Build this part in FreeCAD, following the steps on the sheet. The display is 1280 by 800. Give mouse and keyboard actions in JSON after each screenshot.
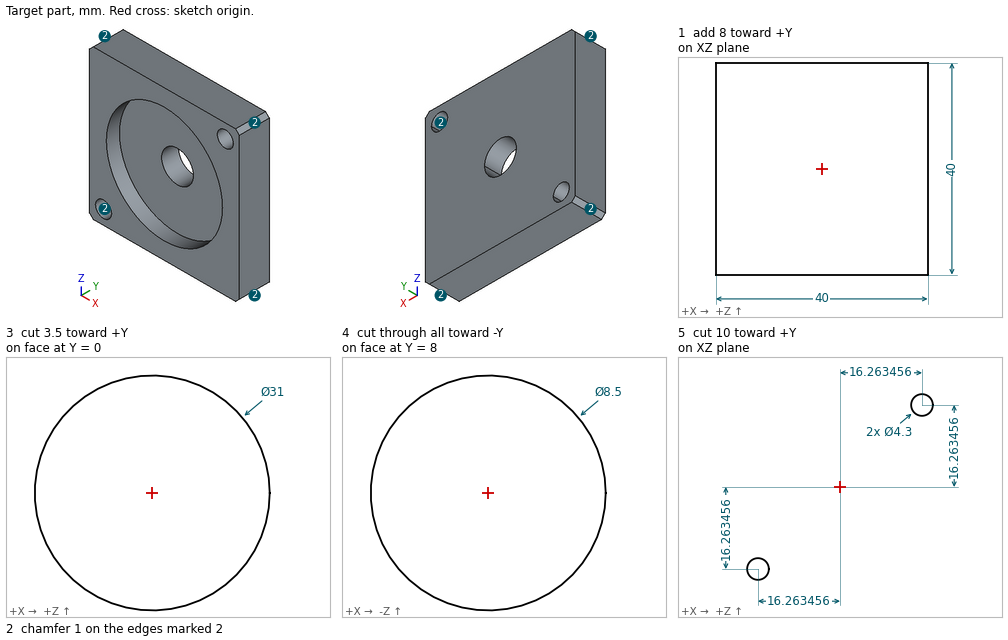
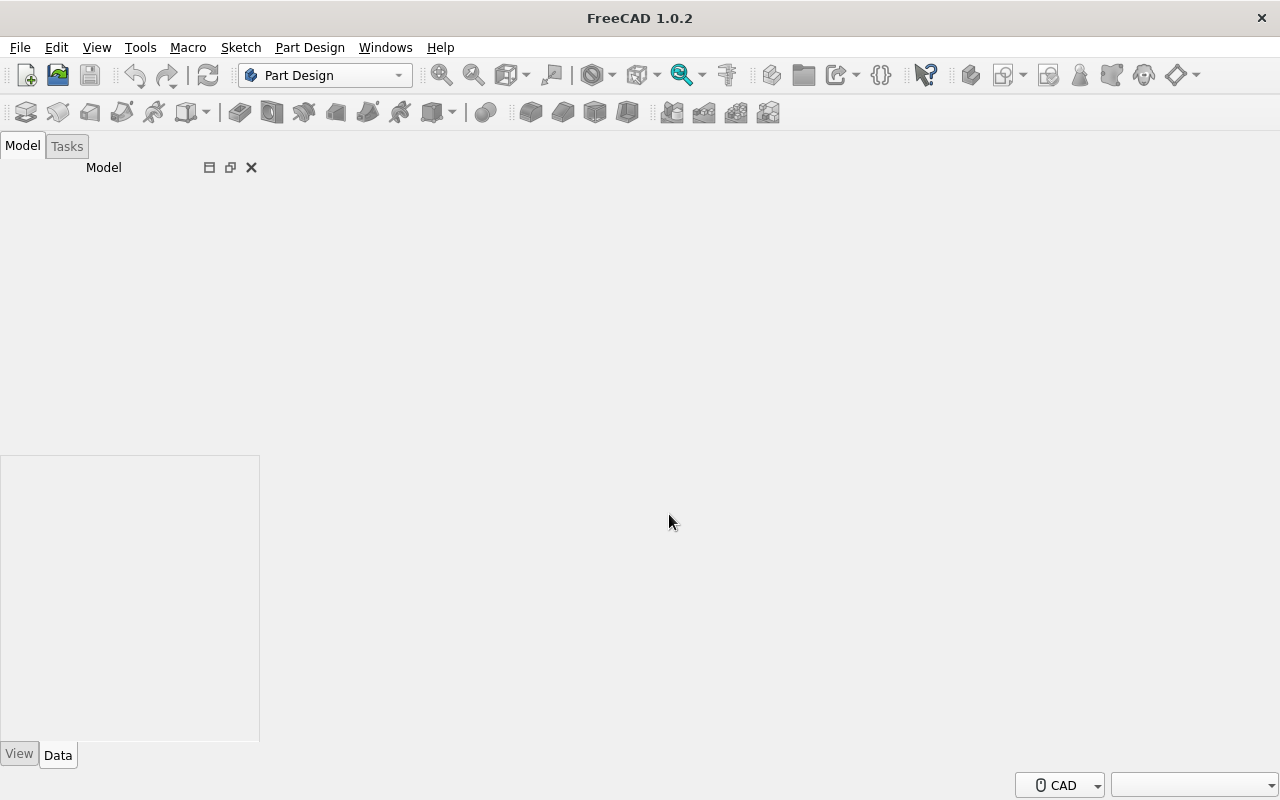
{"action": "left_click", "coordinate": [26, 76]}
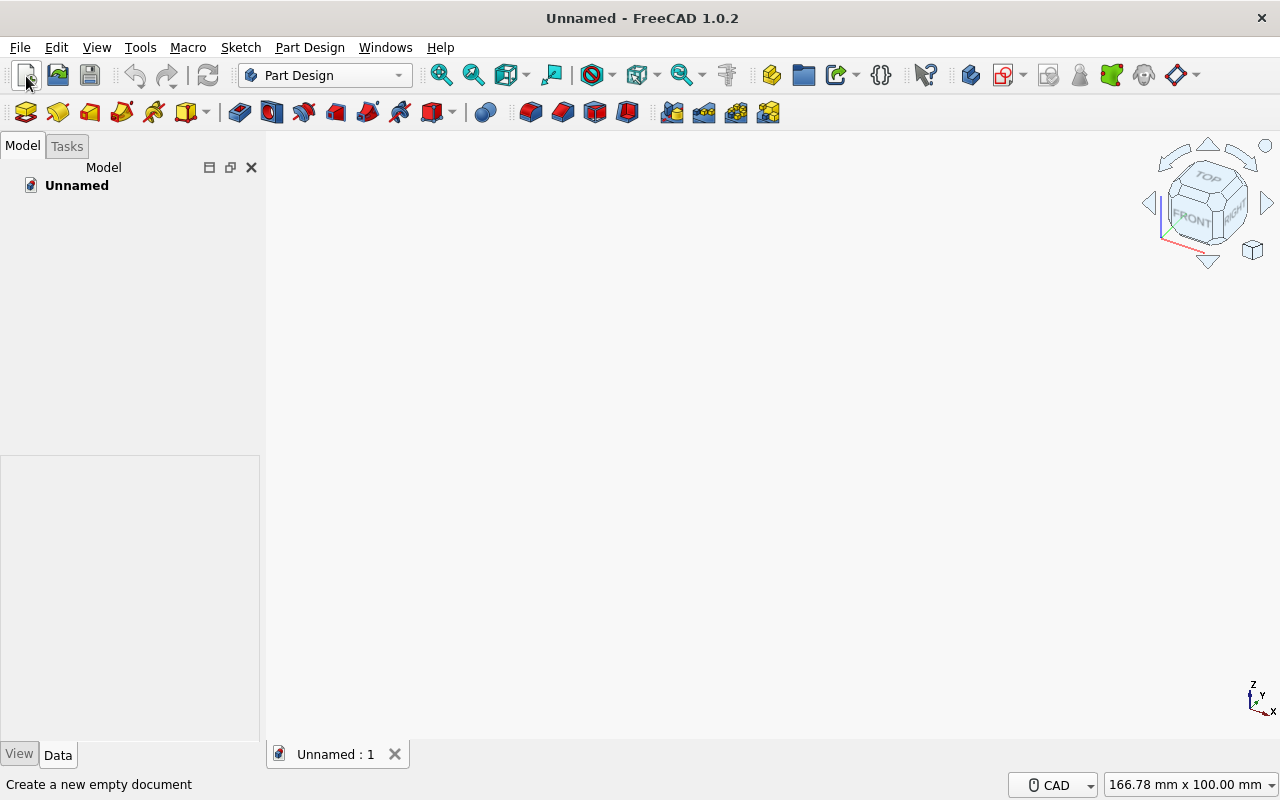
{"action": "left_click", "coordinate": [1004, 76]}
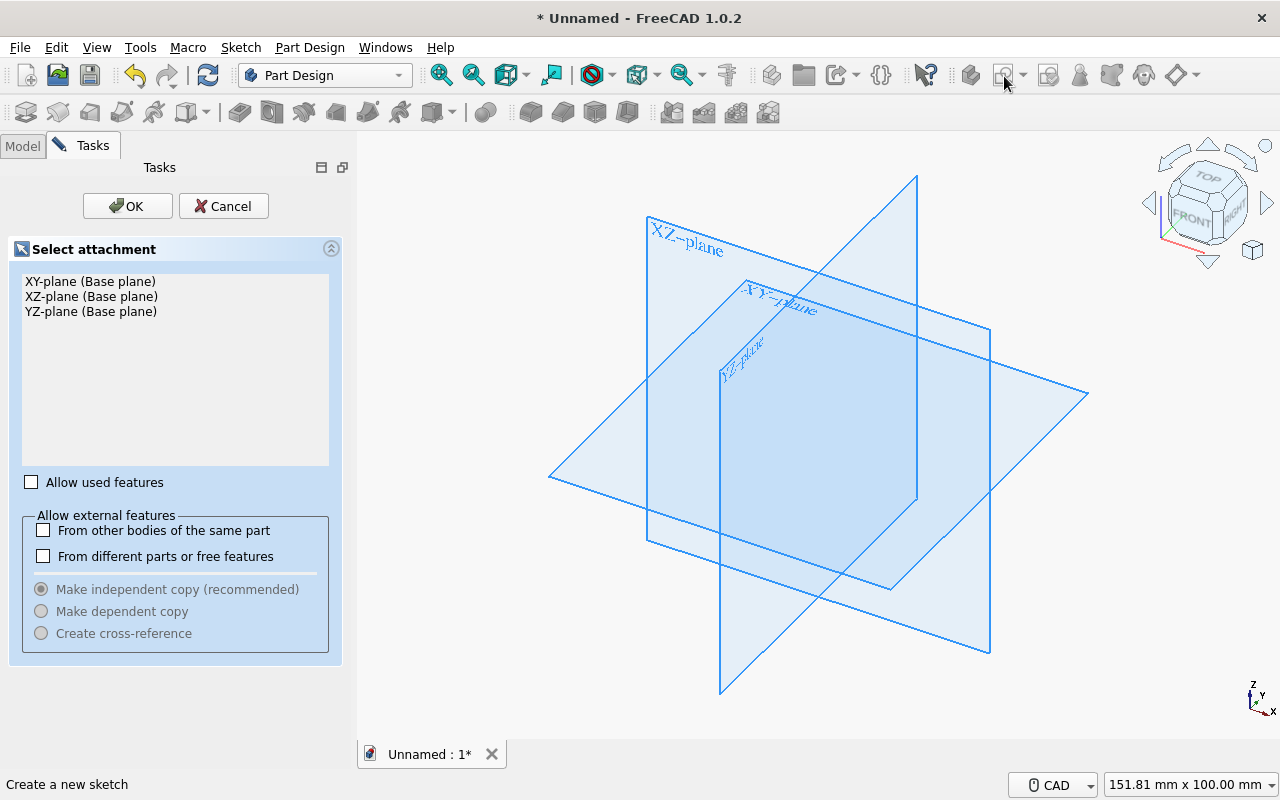
{"action": "left_click", "coordinate": [82, 296]}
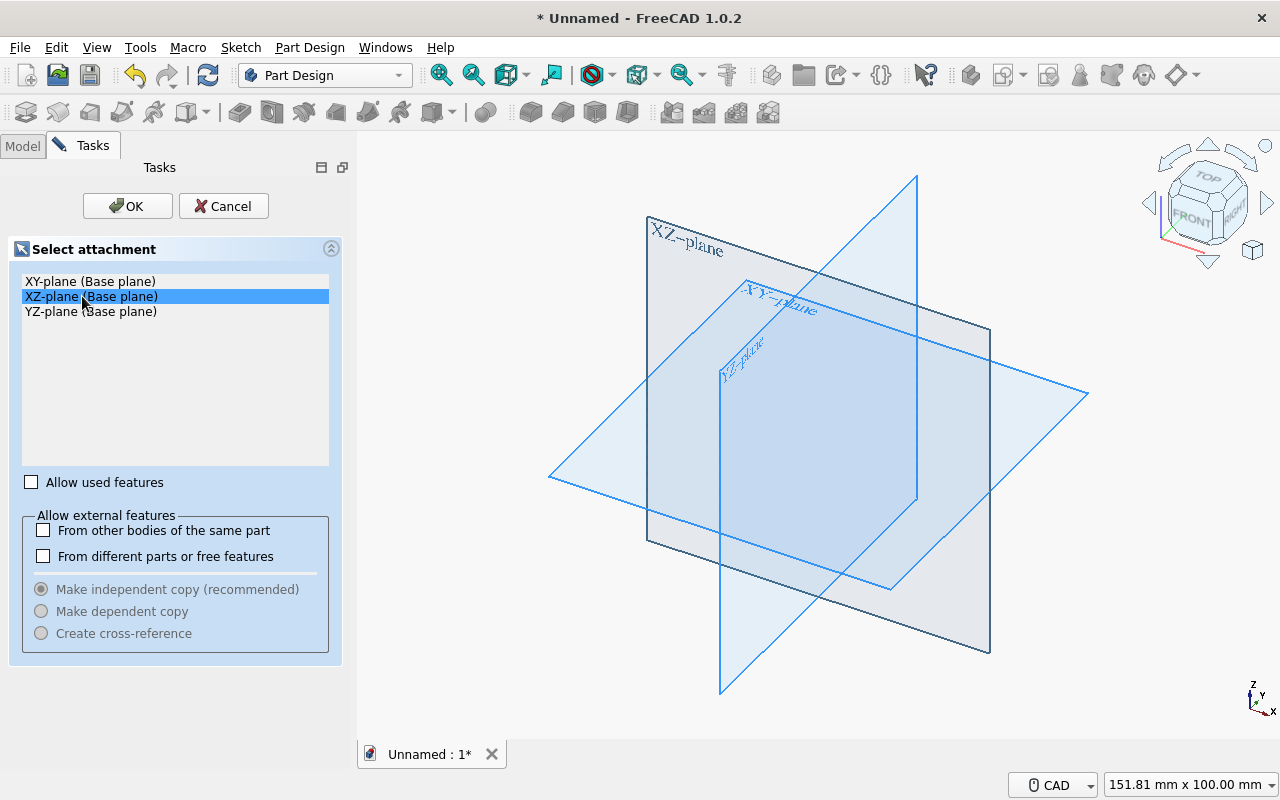
{"action": "left_click", "coordinate": [128, 206]}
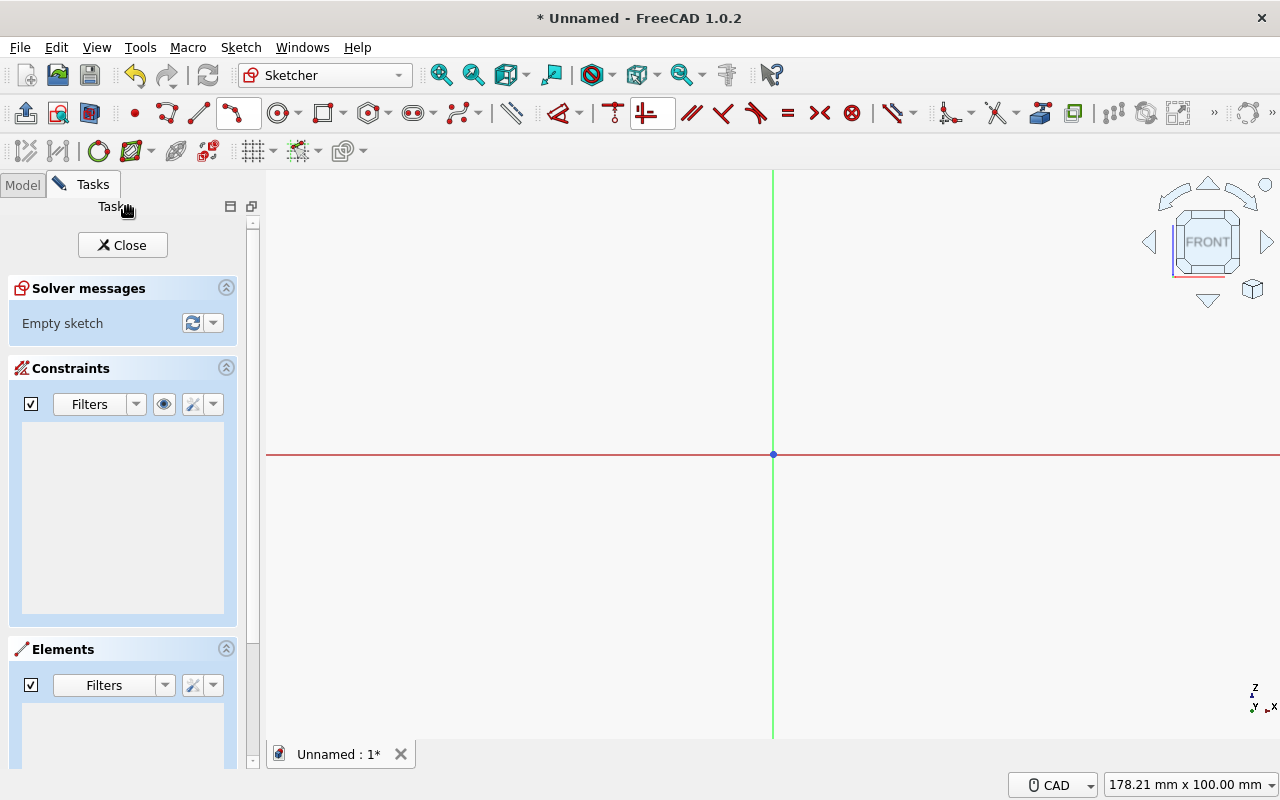
{"action": "scroll", "coordinate": [912, 455], "scroll_direction": "up", "scroll_amount": 2}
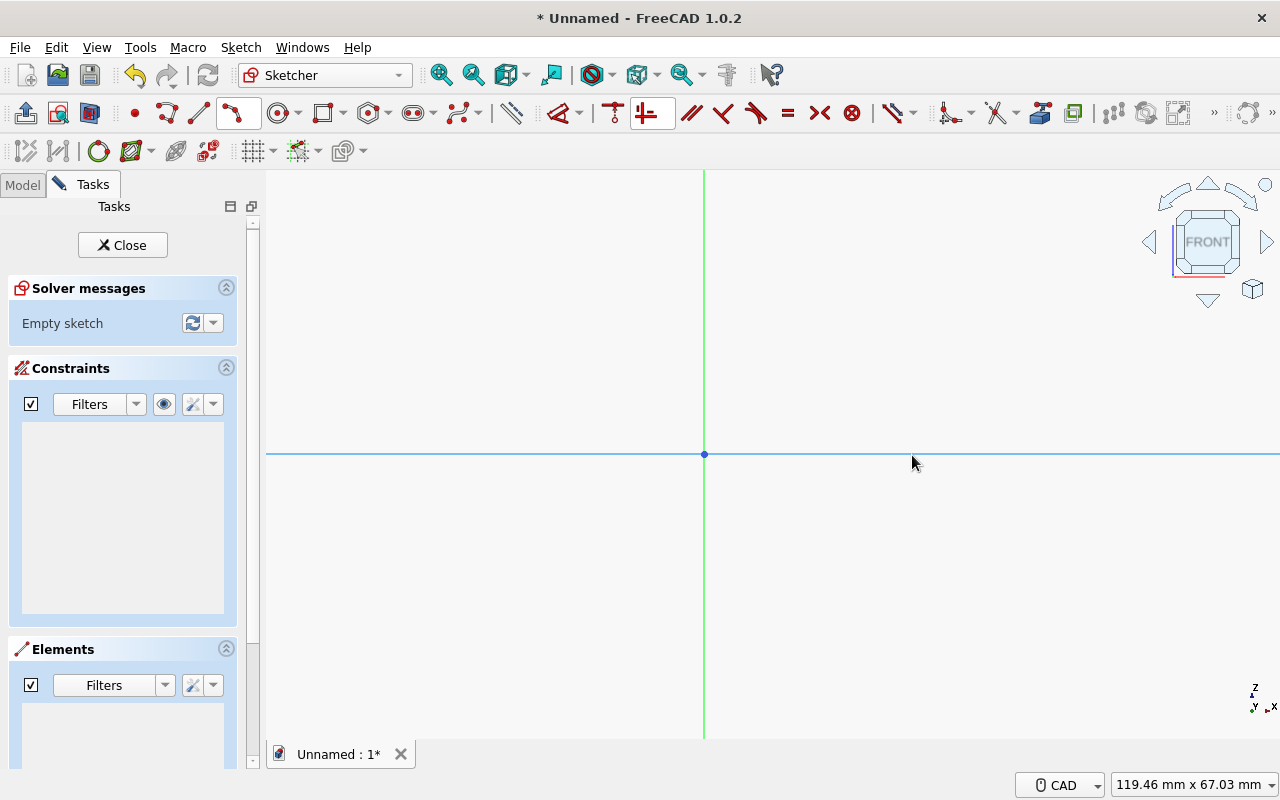
{"action": "left_click", "coordinate": [346, 114]}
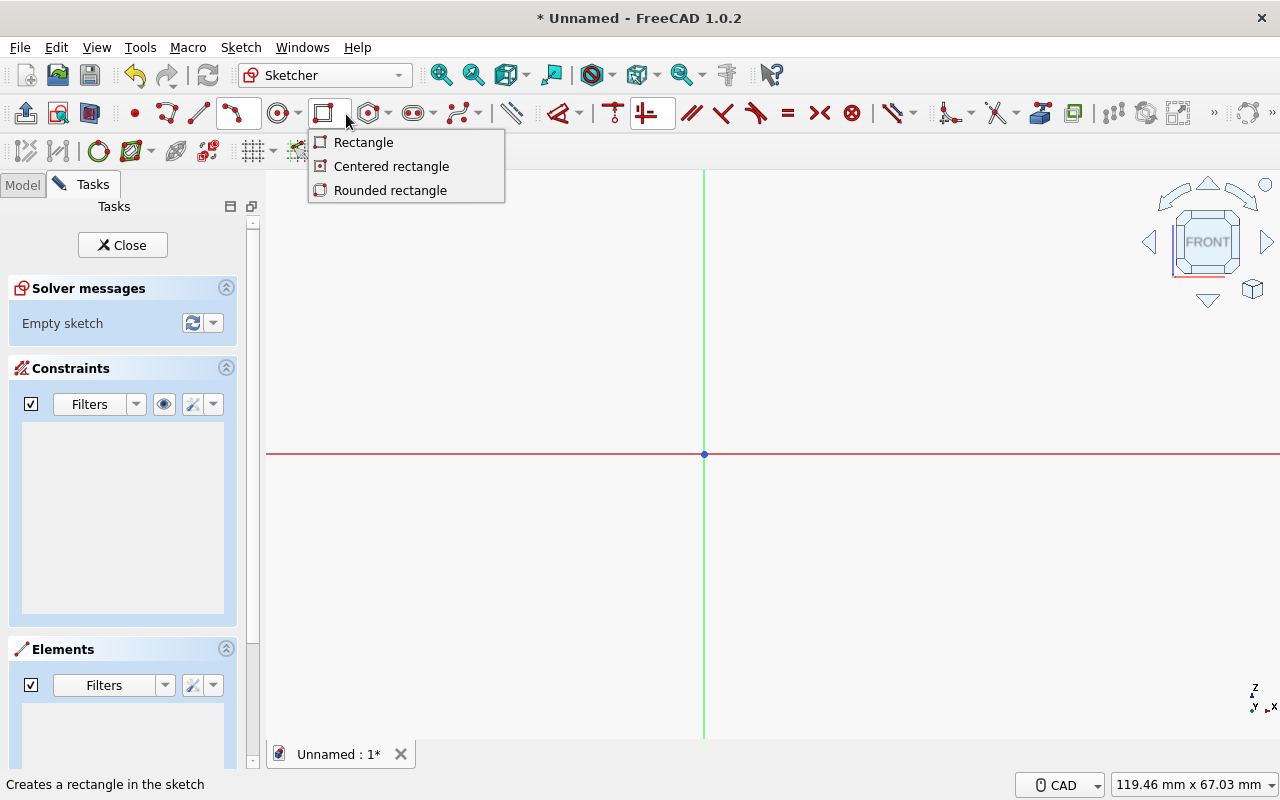
{"action": "left_click", "coordinate": [406, 166]}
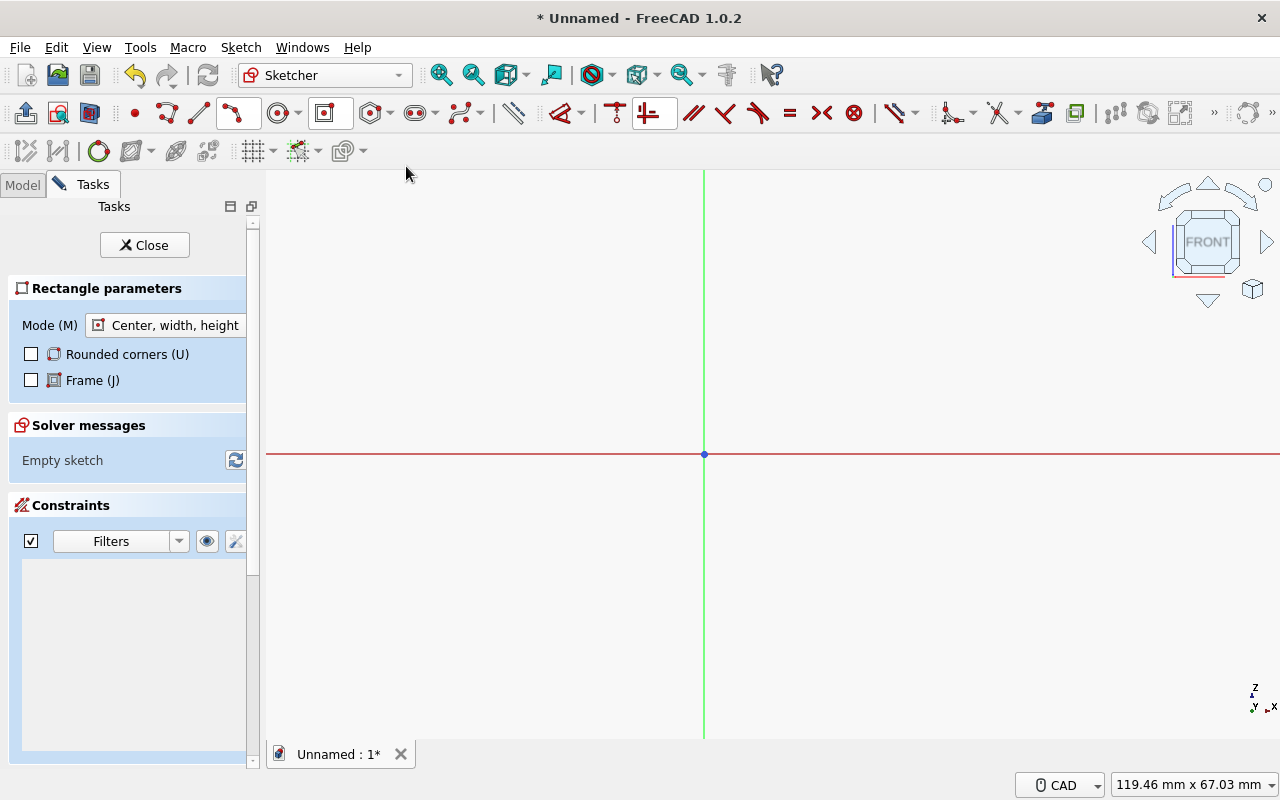
{"action": "left_click", "coordinate": [704, 454]}
{"action": "left_click", "coordinate": [874, 284]}
{"action": "key", "text": "Escape"}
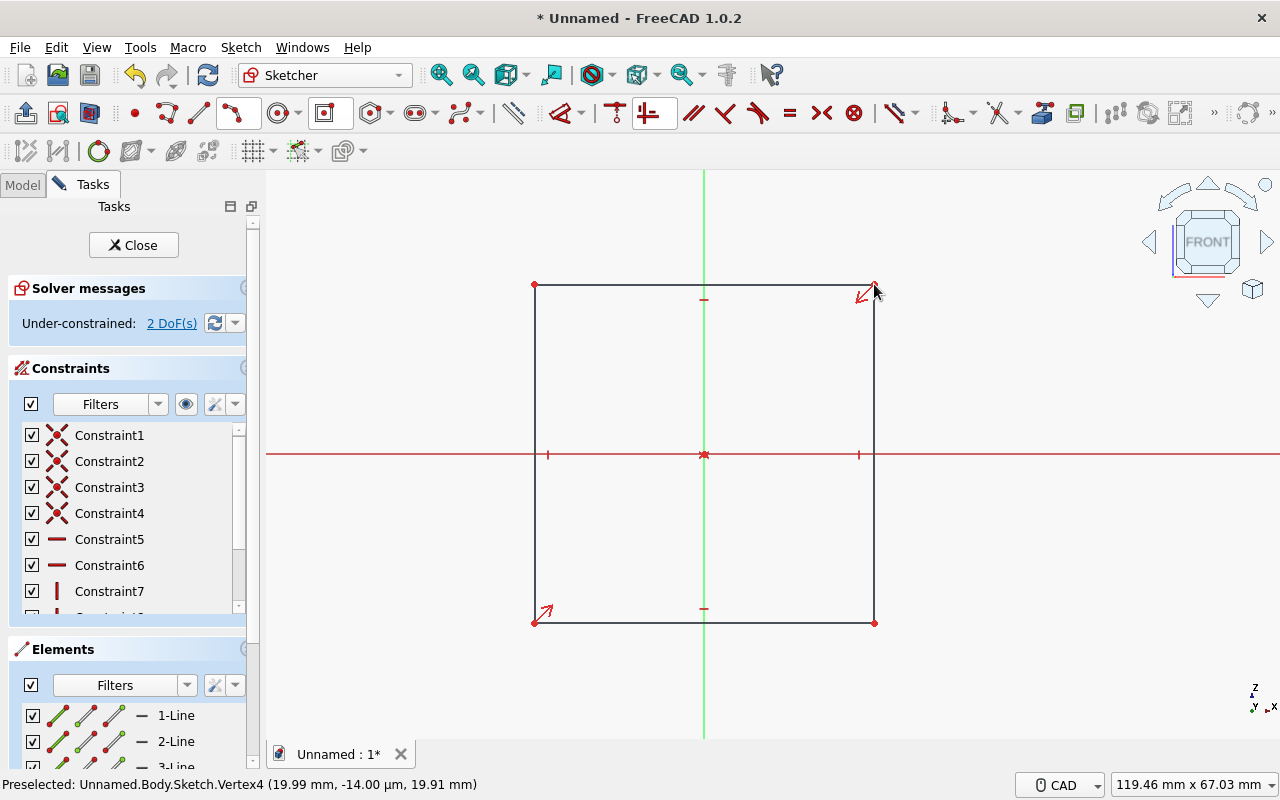
{"action": "left_click", "coordinate": [560, 114]}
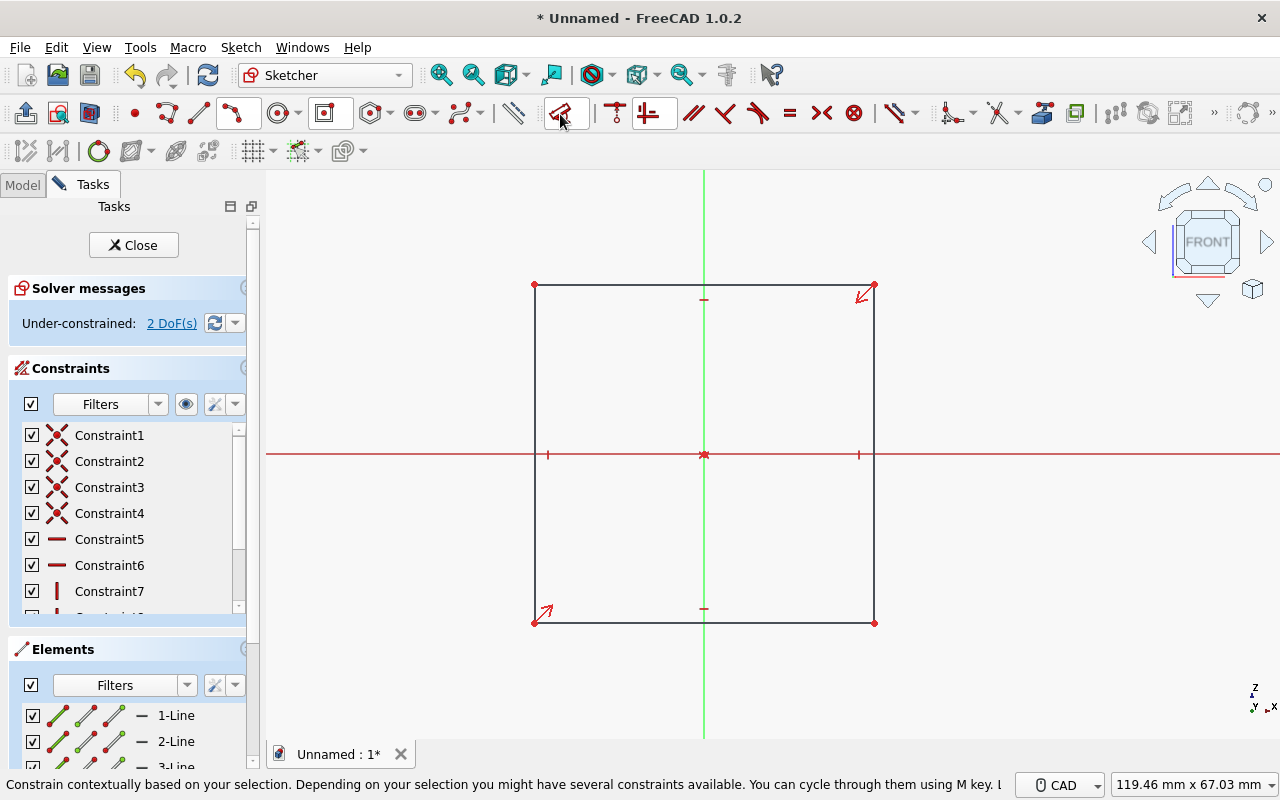
{"action": "left_click", "coordinate": [636, 623]}
{"action": "left_click", "coordinate": [626, 657]}